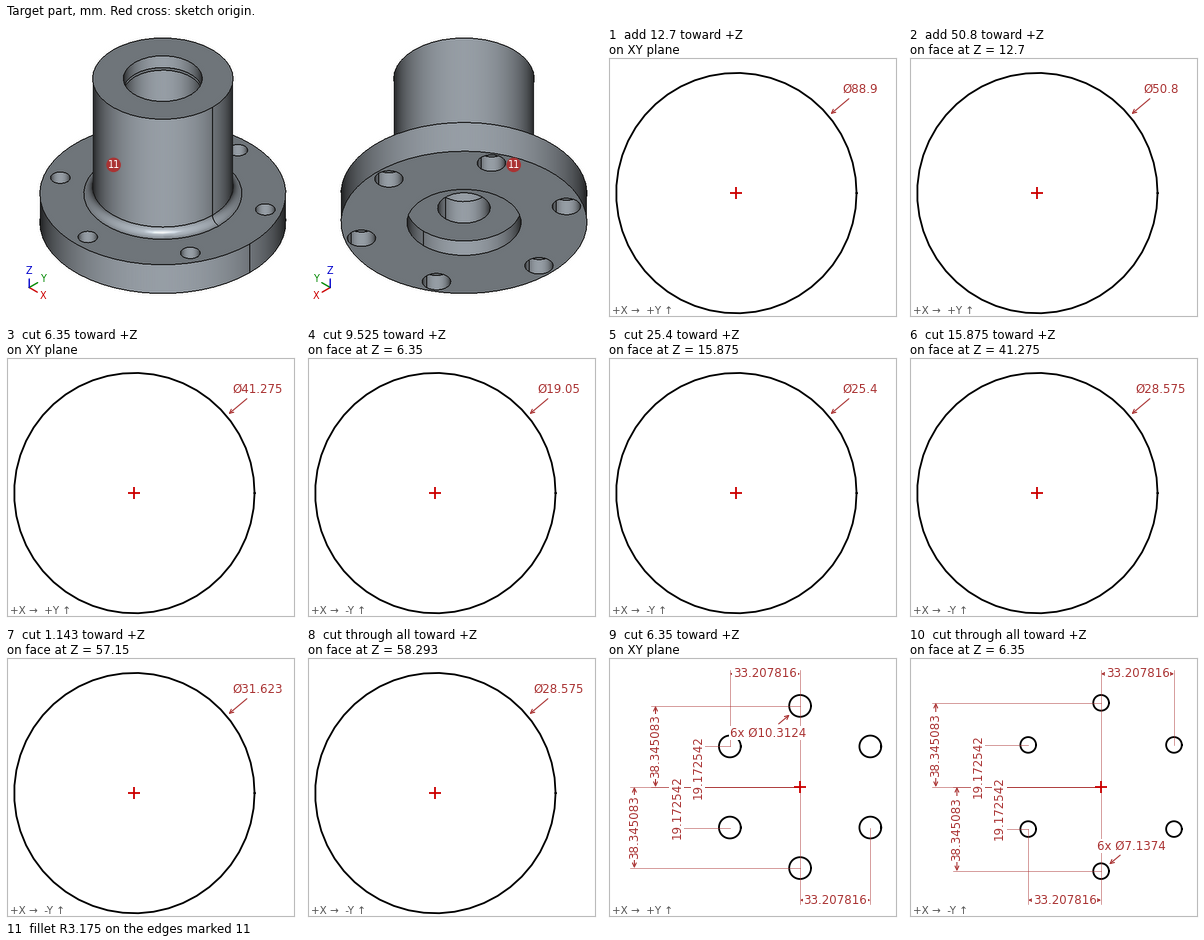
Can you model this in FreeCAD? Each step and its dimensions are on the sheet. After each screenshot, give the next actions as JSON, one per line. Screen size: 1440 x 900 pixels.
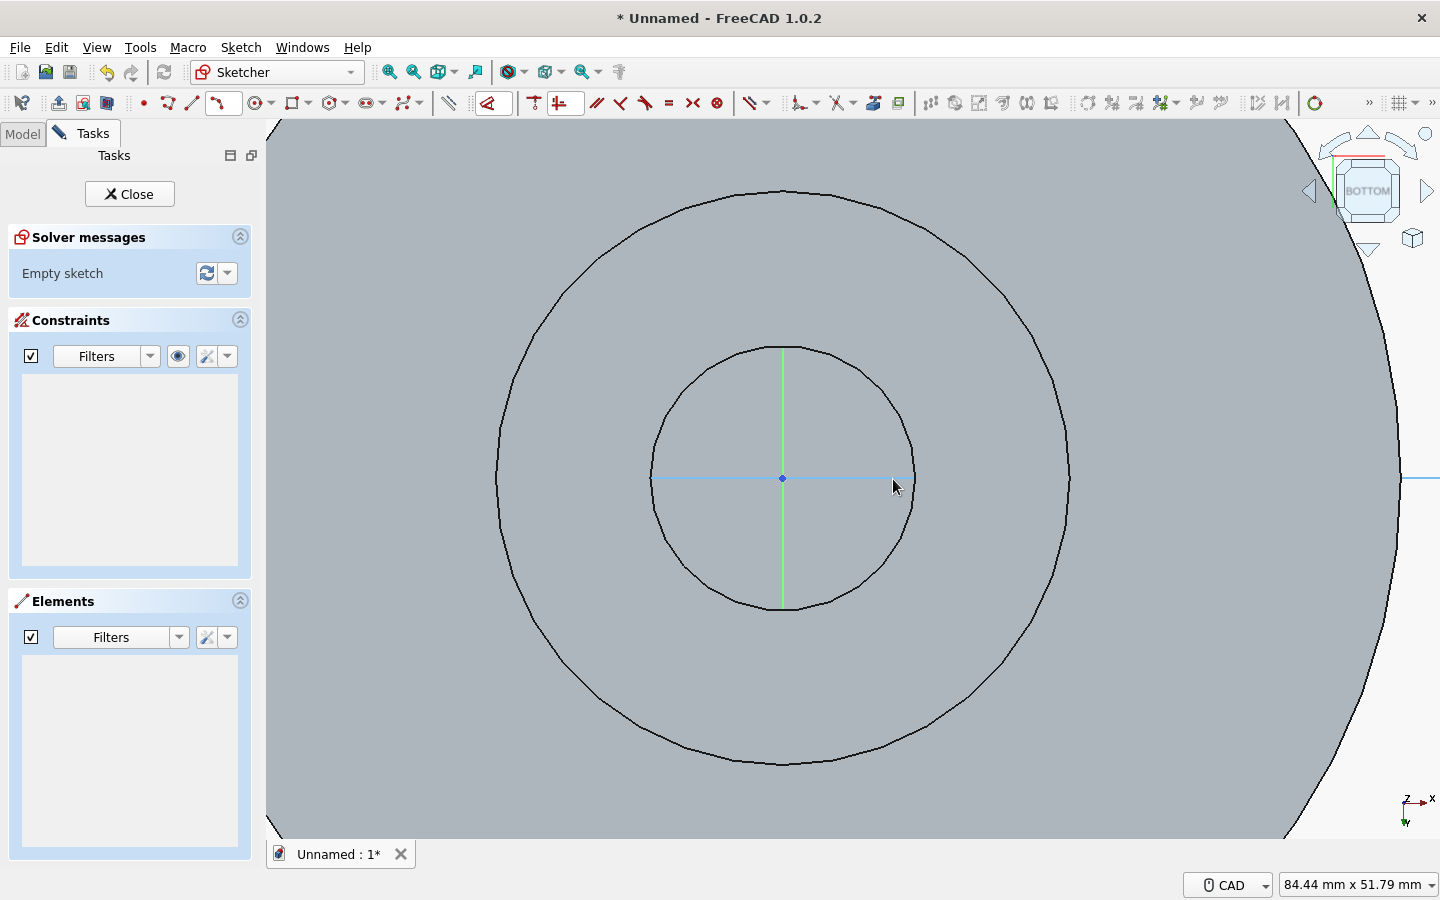
{"action": "left_click", "coordinate": [256, 104]}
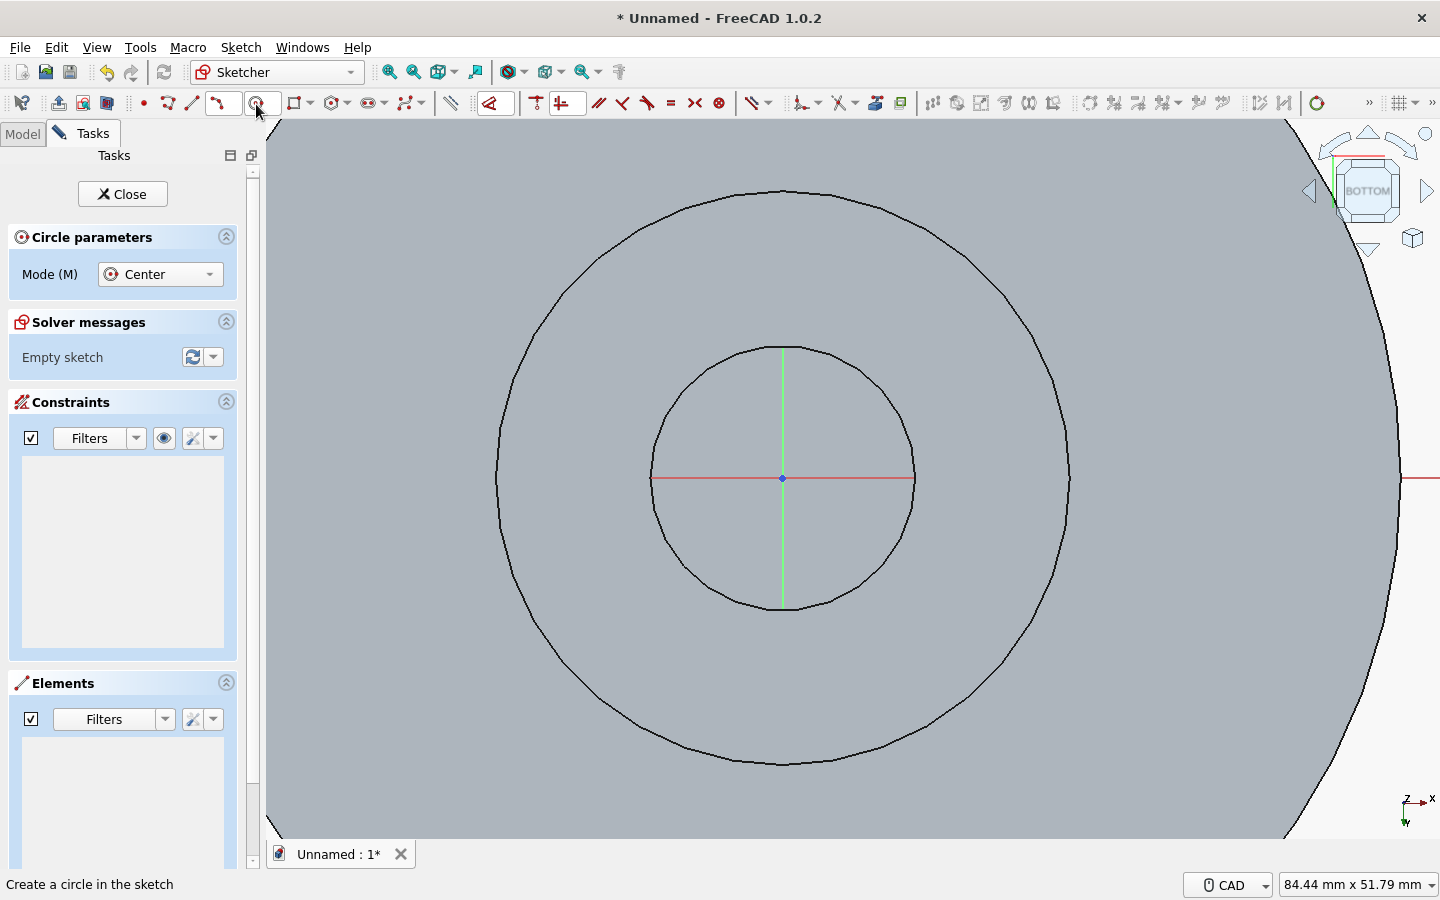
{"action": "left_click", "coordinate": [783, 478]}
{"action": "mouse_move", "coordinate": [938, 323]}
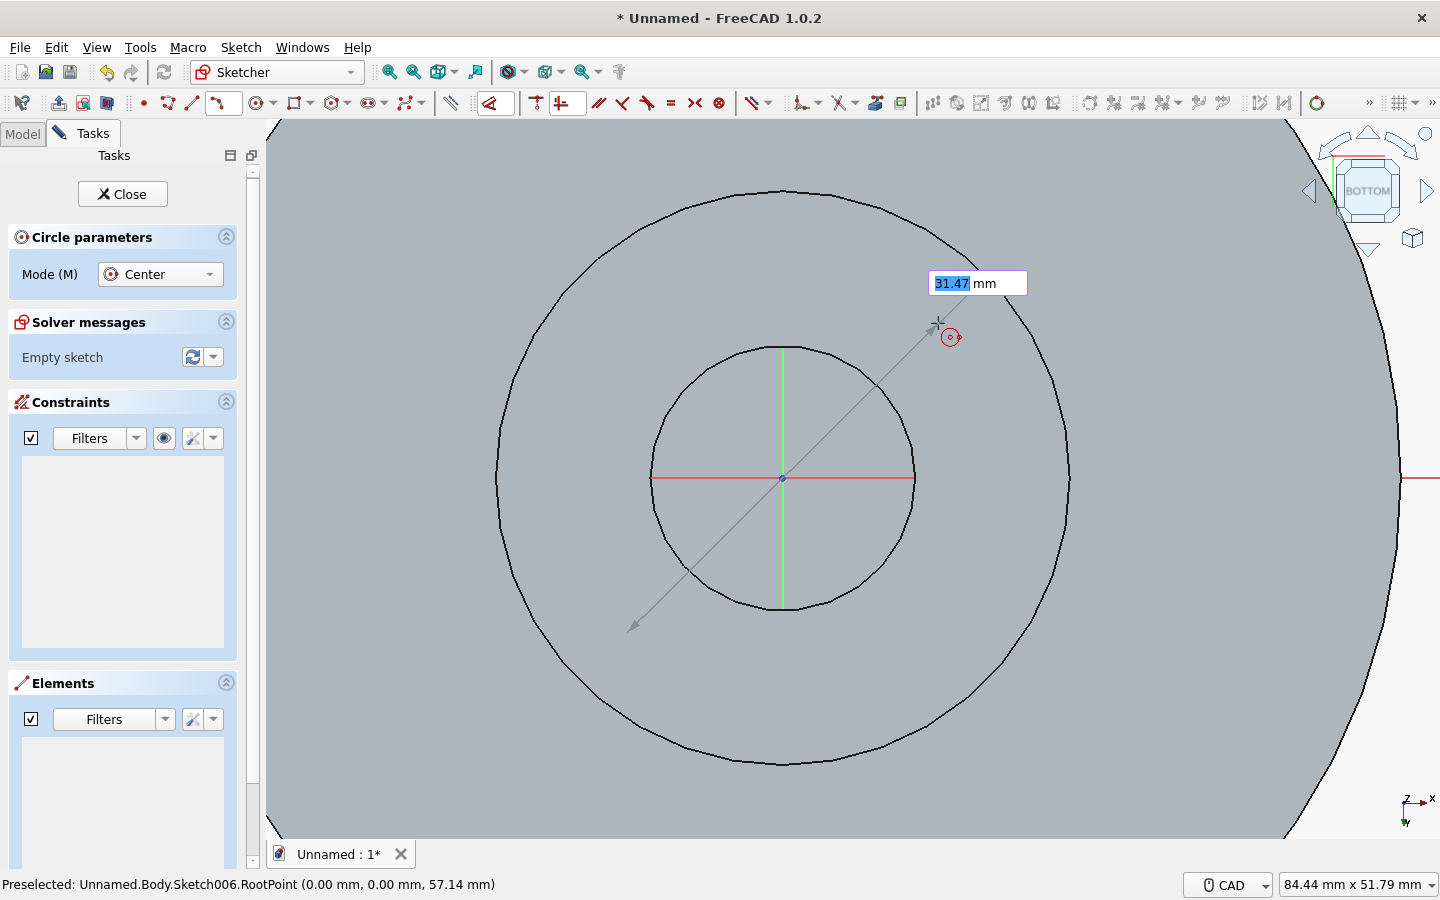
{"action": "type", "text": "31.623"}
{"action": "key", "text": "Return"}
{"action": "key", "text": "Escape"}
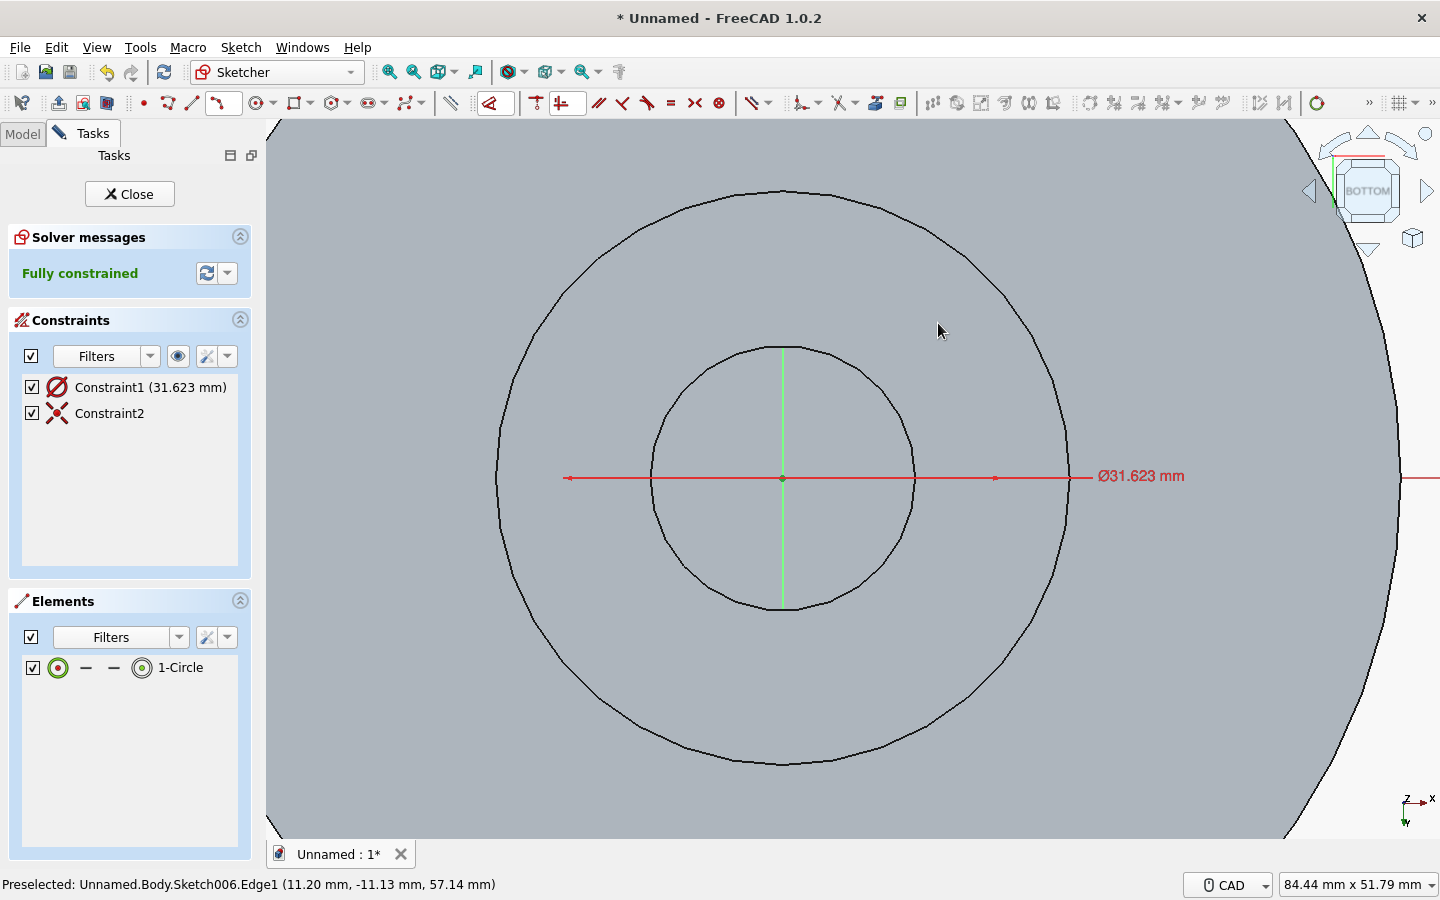
{"action": "left_click", "coordinate": [130, 194]}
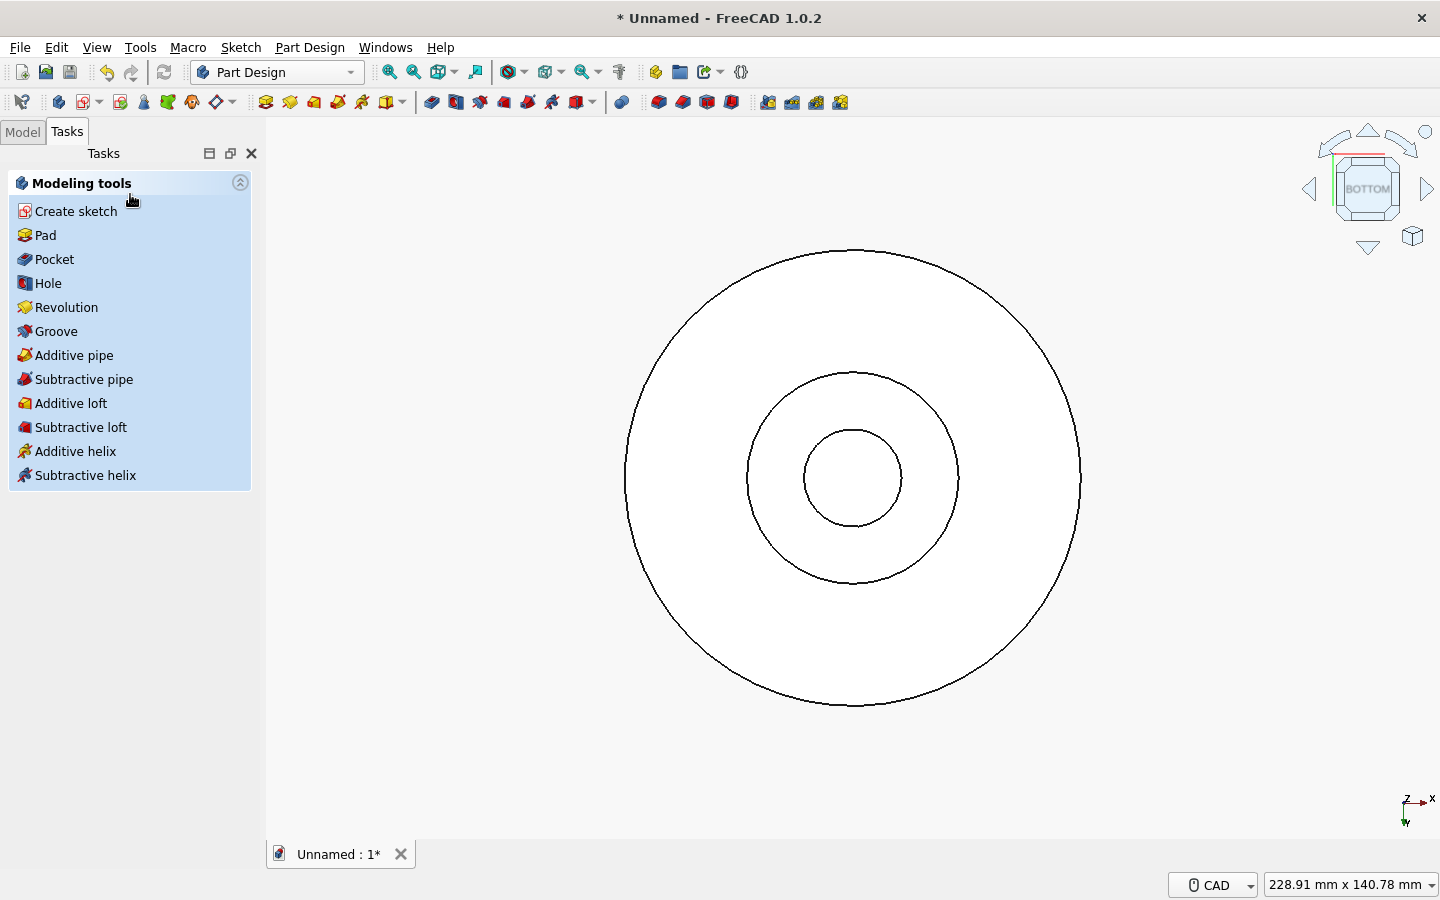
{"action": "left_click", "coordinate": [432, 102]}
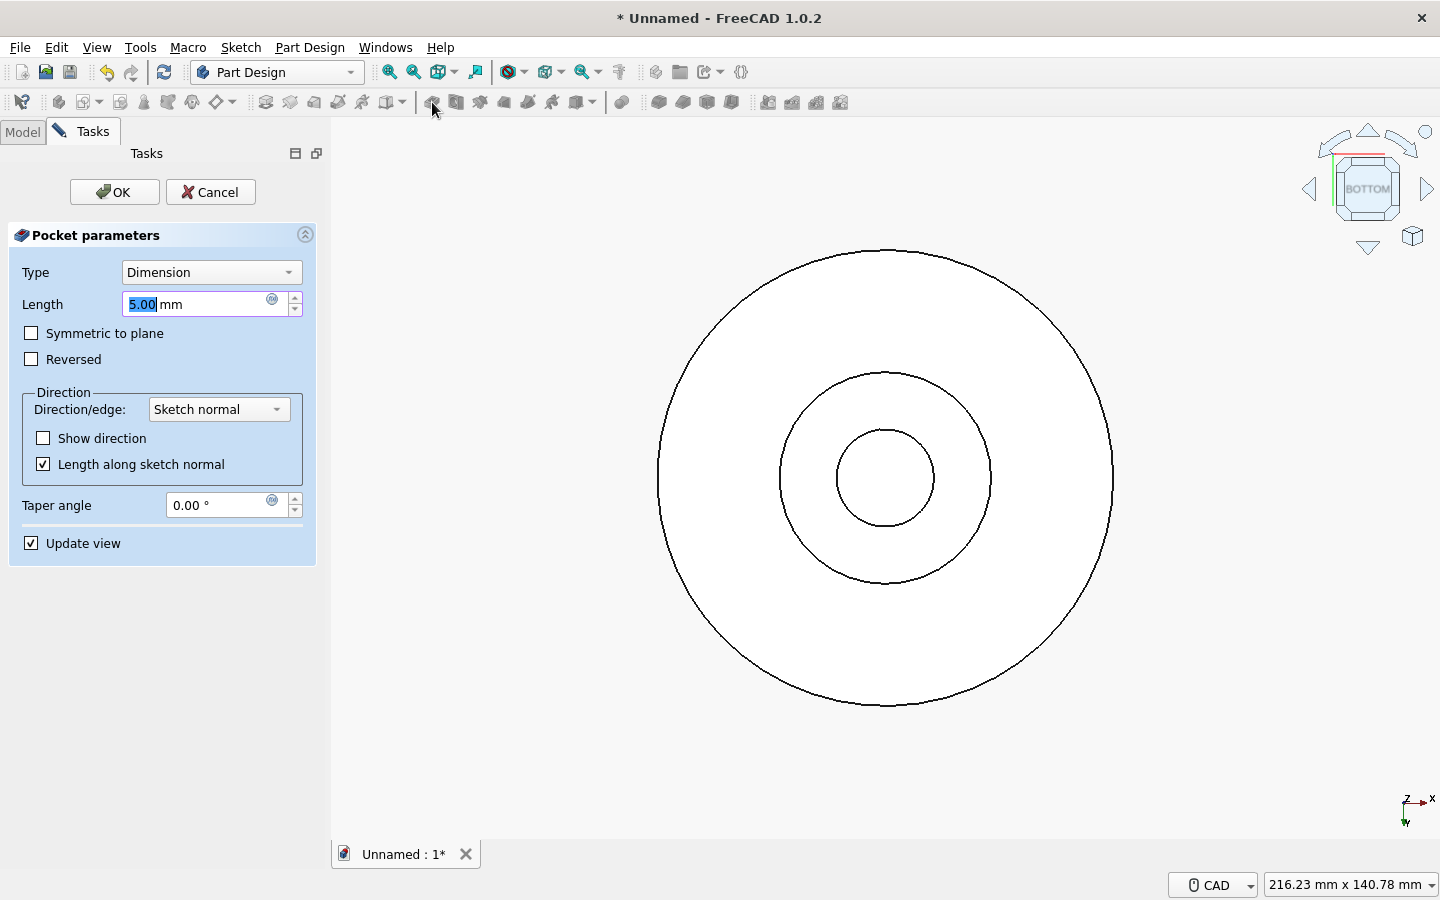
{"action": "type", "text": "1.143"}
{"action": "key", "text": "Tab"}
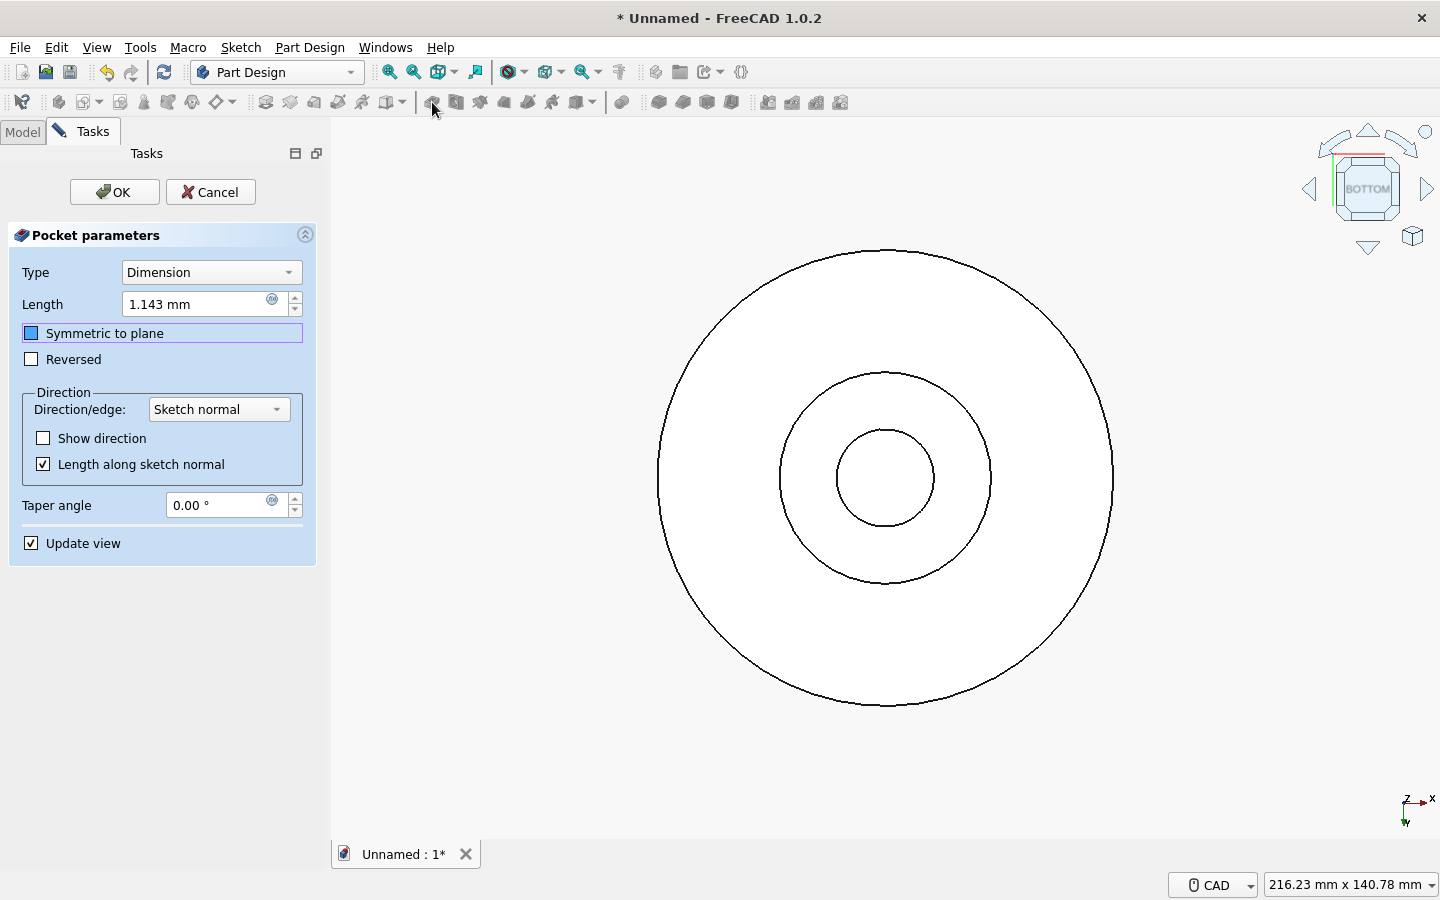
{"action": "left_click", "coordinate": [115, 192]}